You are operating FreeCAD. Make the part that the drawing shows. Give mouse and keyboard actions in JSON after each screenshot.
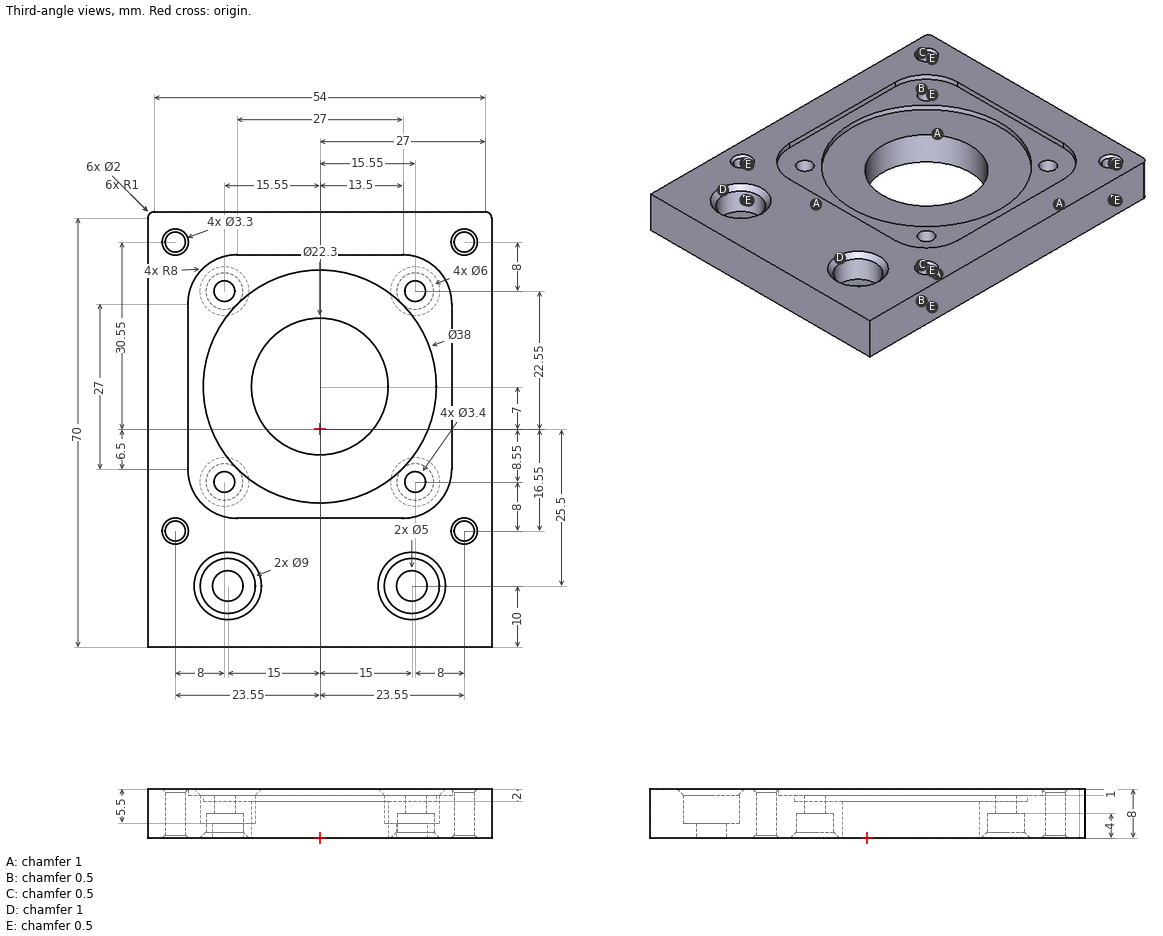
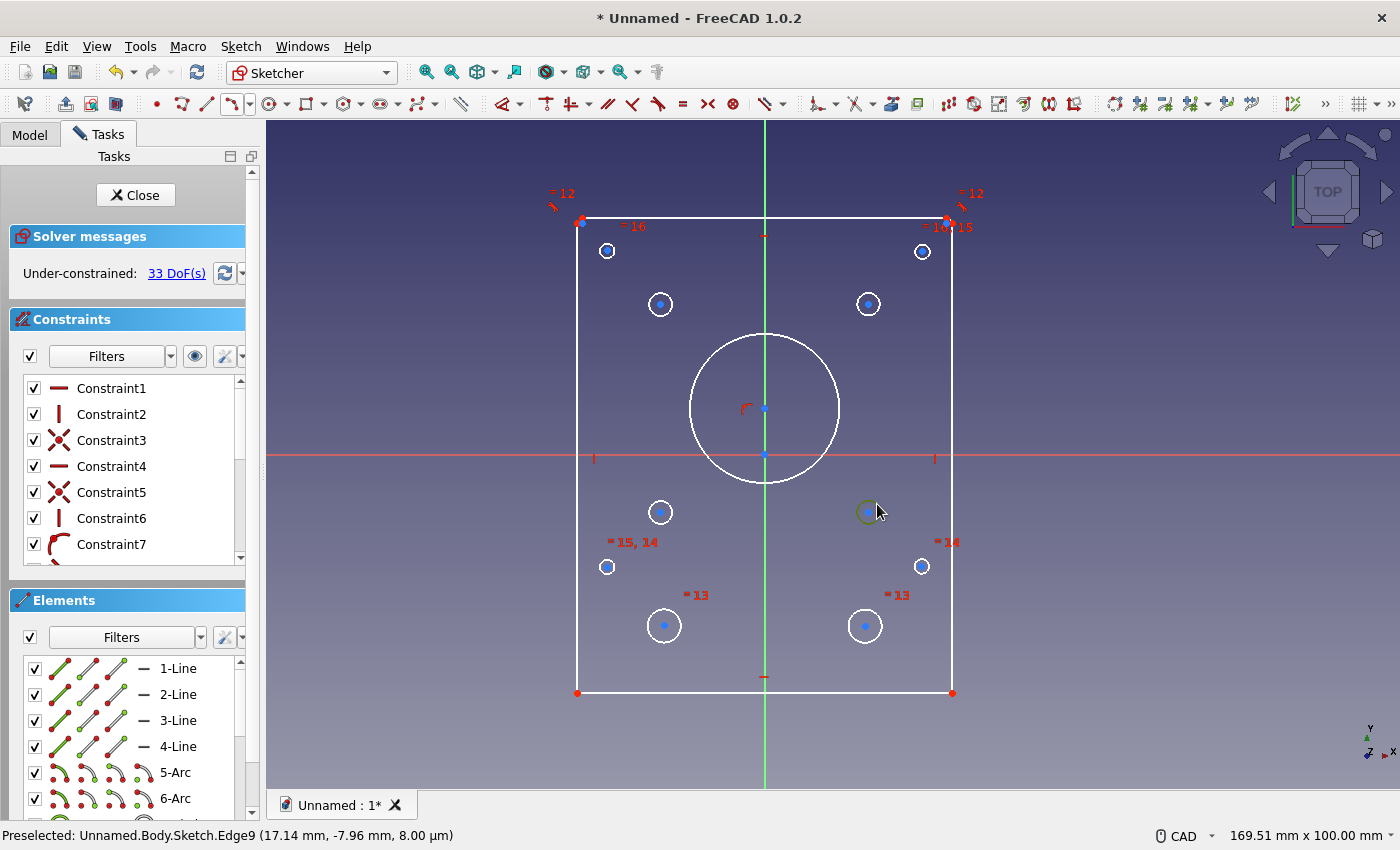
{"action": "left_click", "coordinate": [669, 504]}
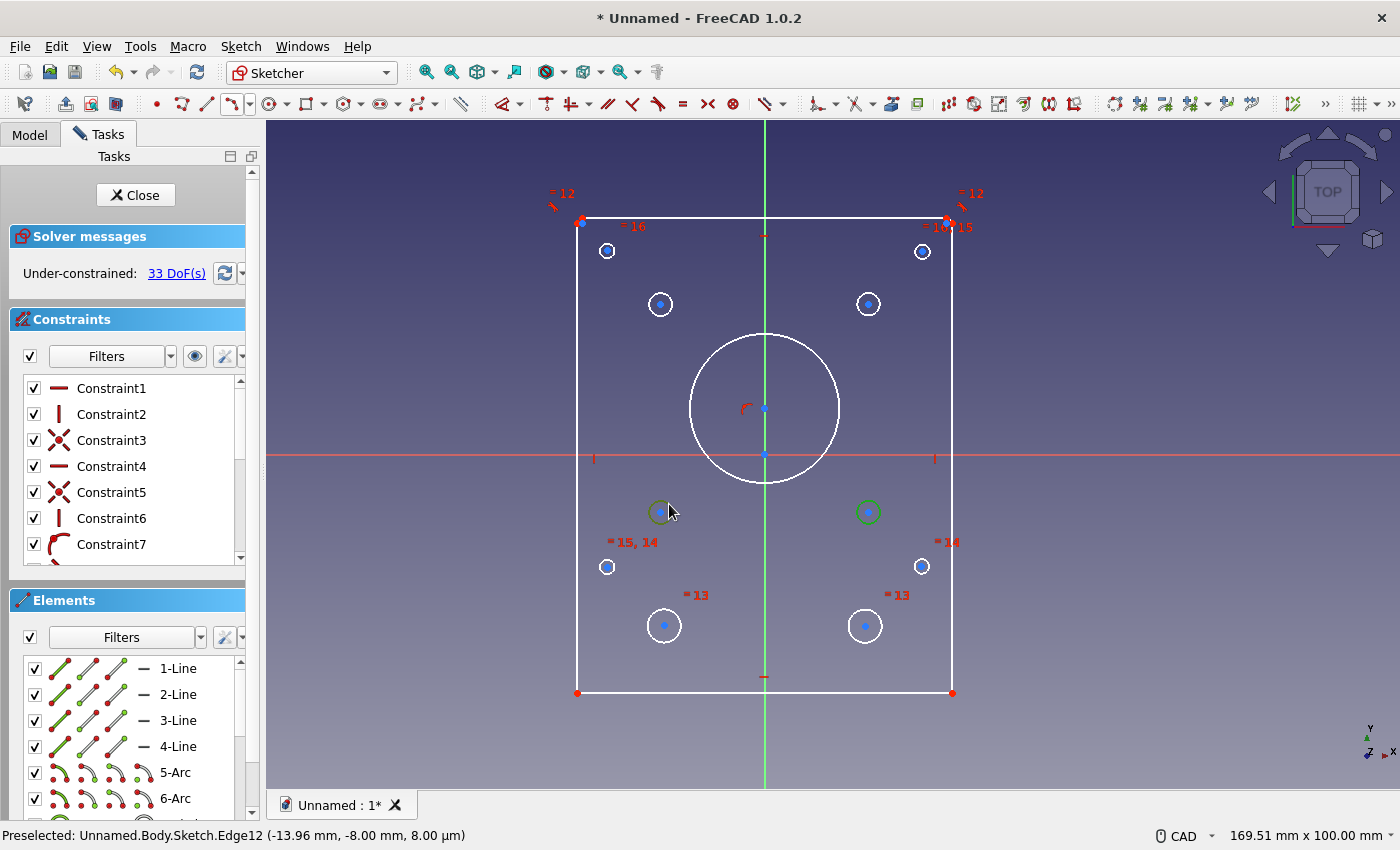
{"action": "scroll", "coordinate": [876, 296], "scroll_direction": "up", "scroll_amount": 2}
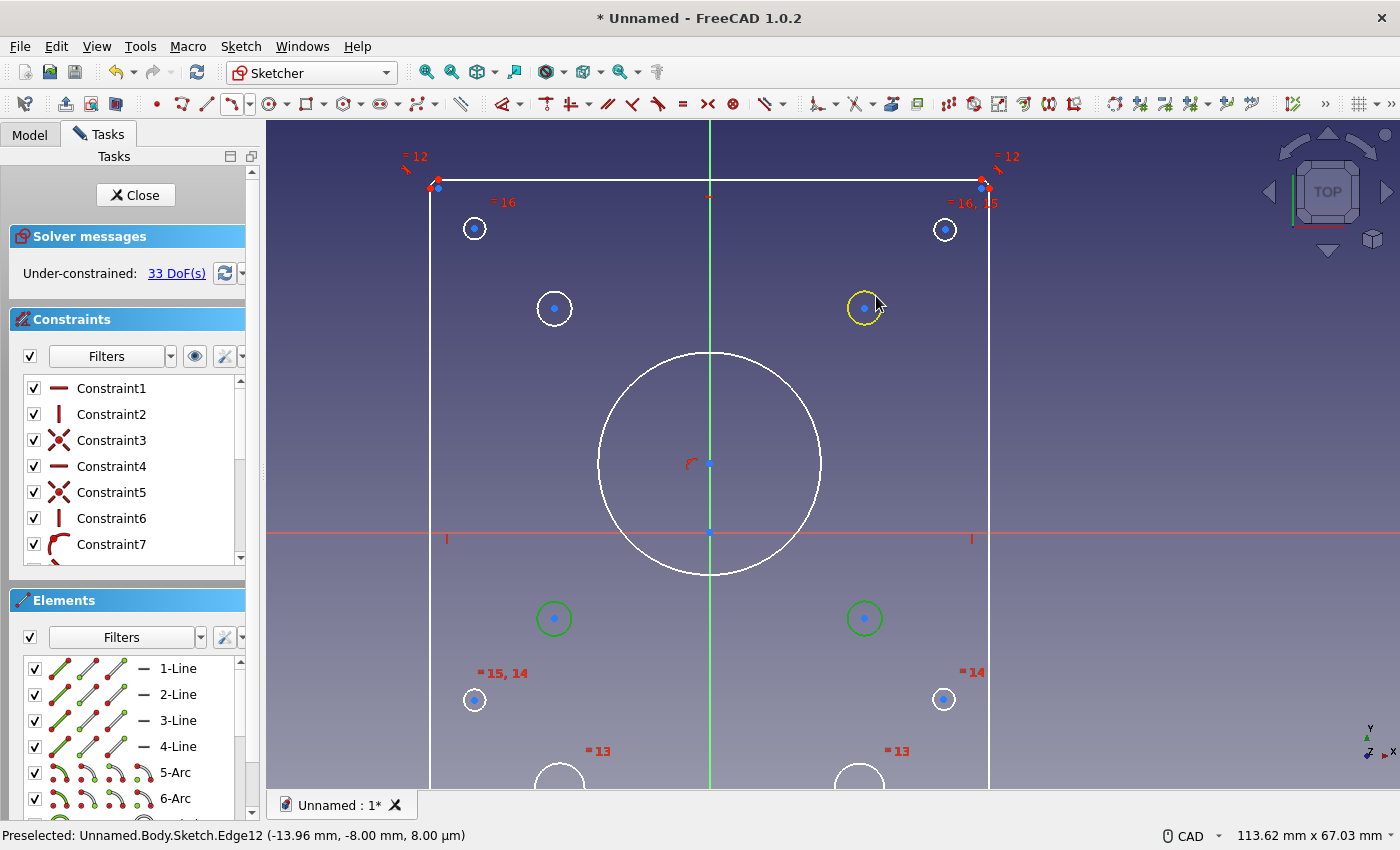
{"action": "left_click", "coordinate": [876, 296]}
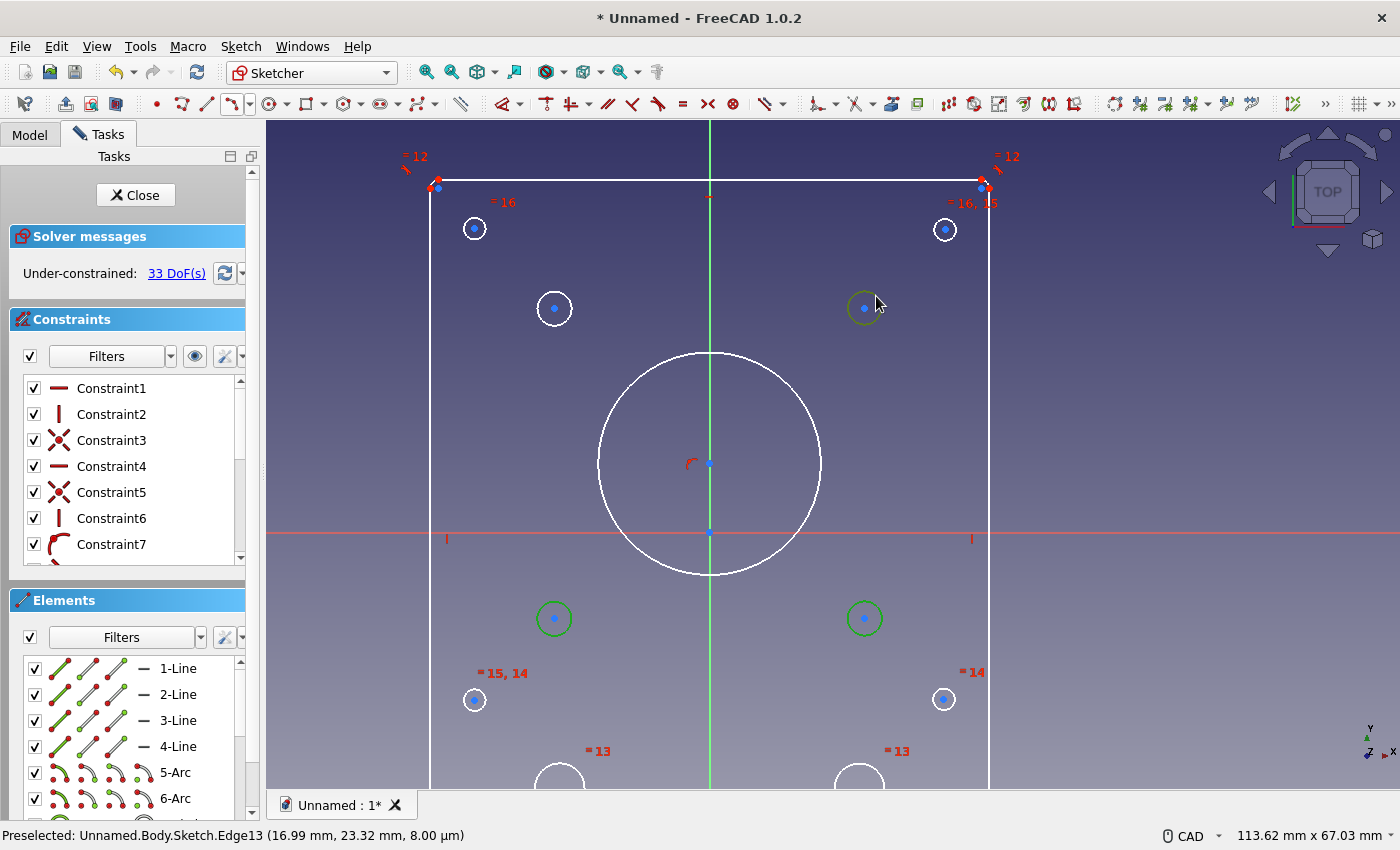
{"action": "left_click", "coordinate": [567, 297]}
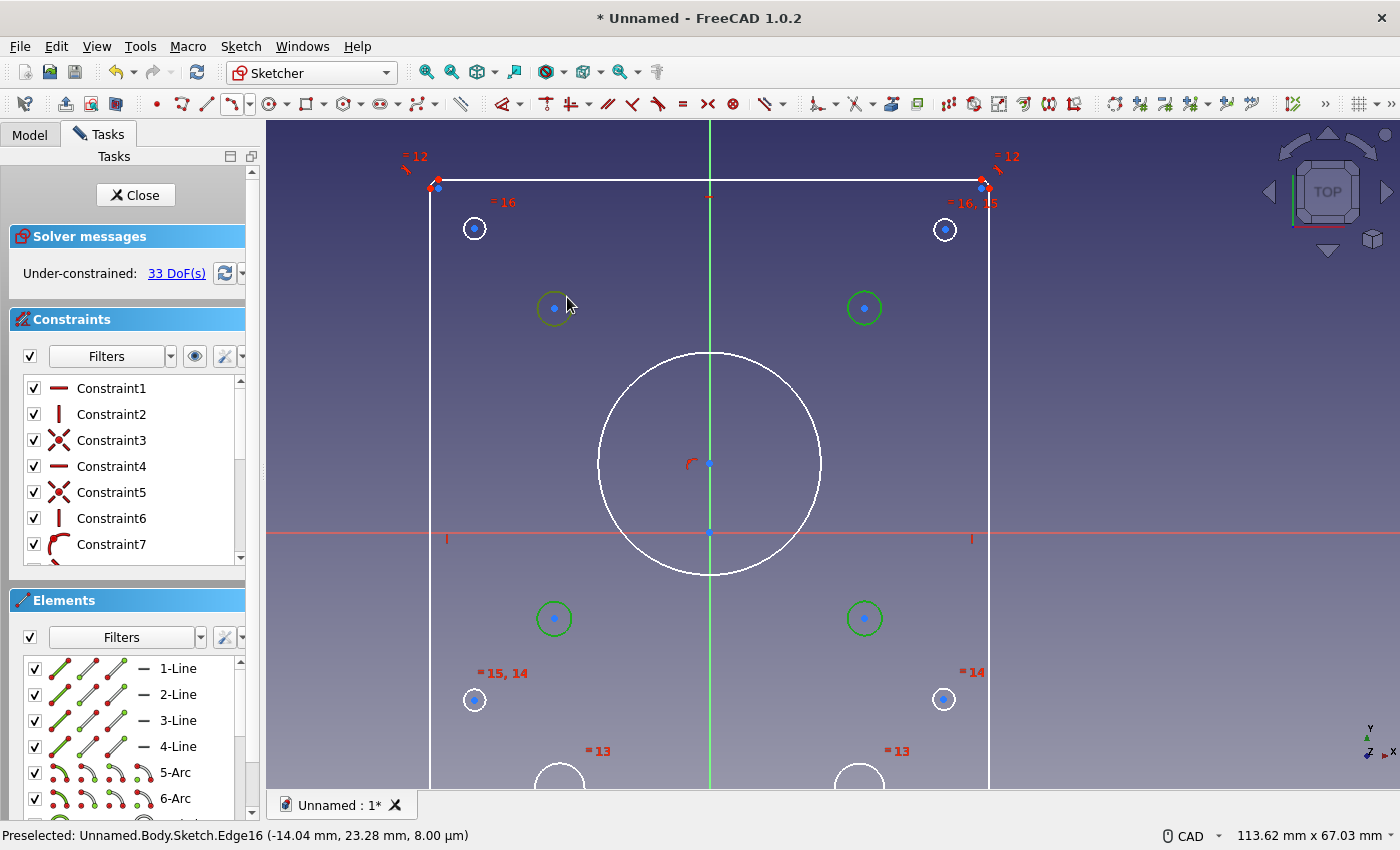
{"action": "left_click", "coordinate": [683, 104]}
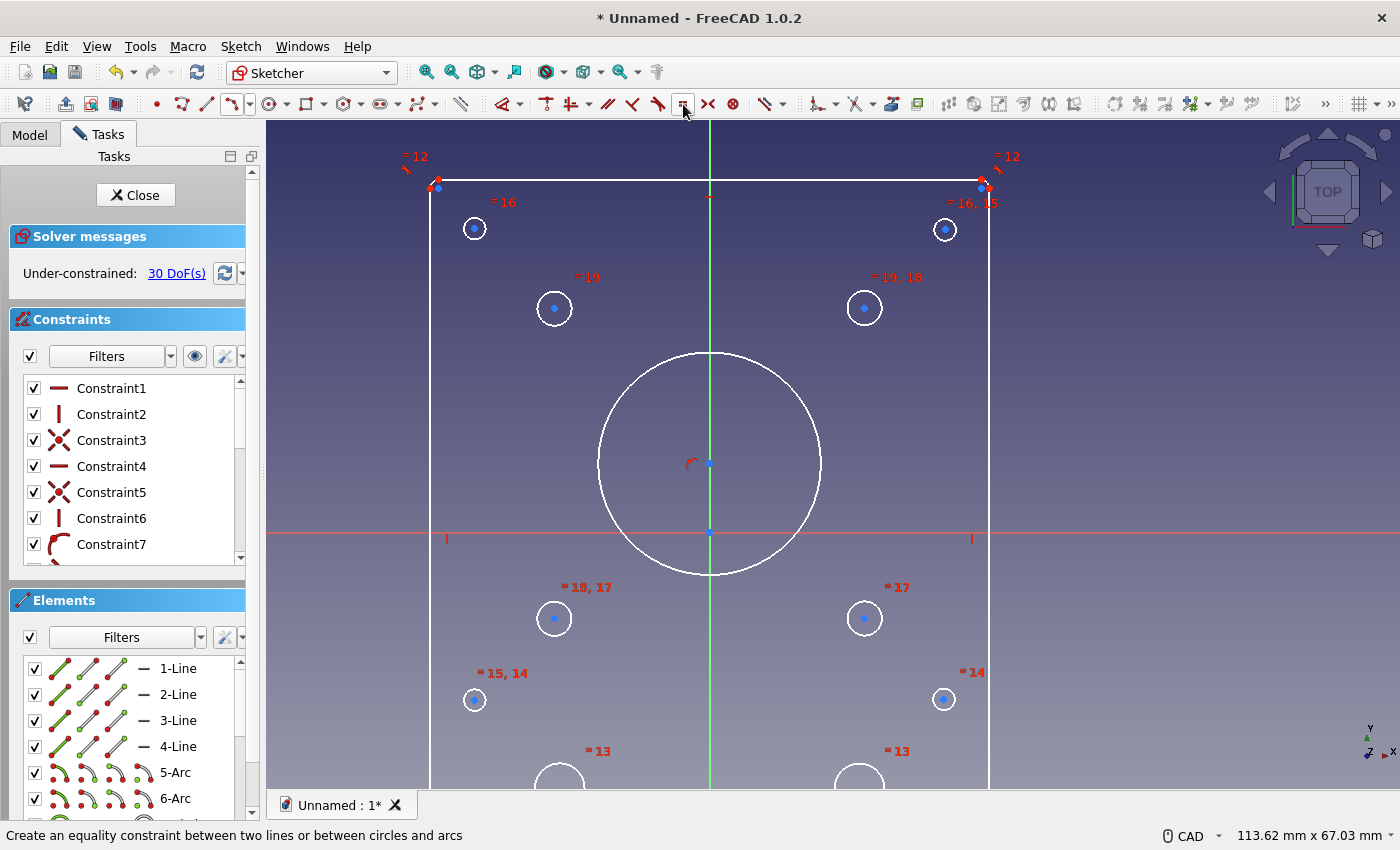
{"action": "key", "text": "d"}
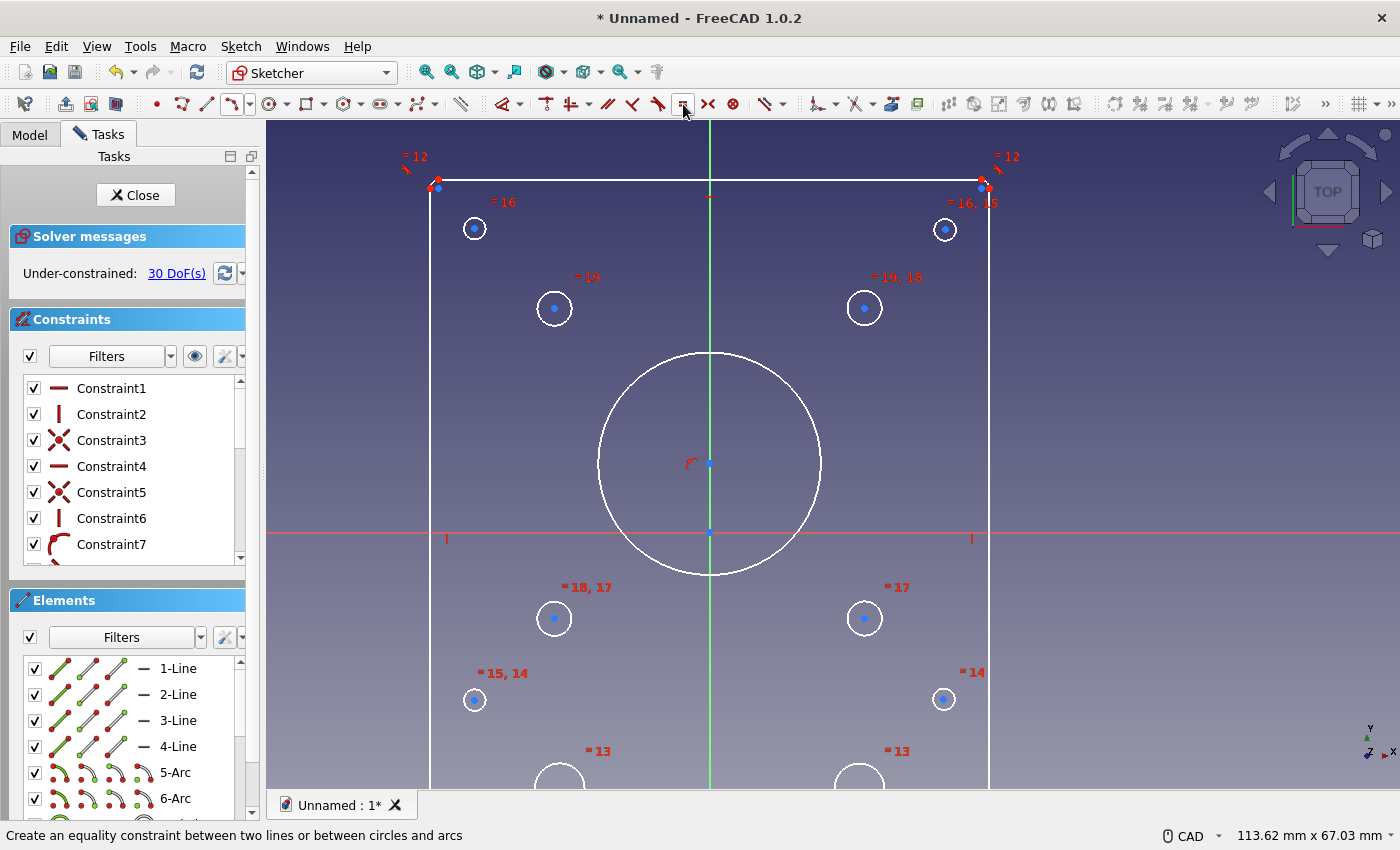
{"action": "scroll", "coordinate": [433, 182], "scroll_direction": "up", "scroll_amount": 7}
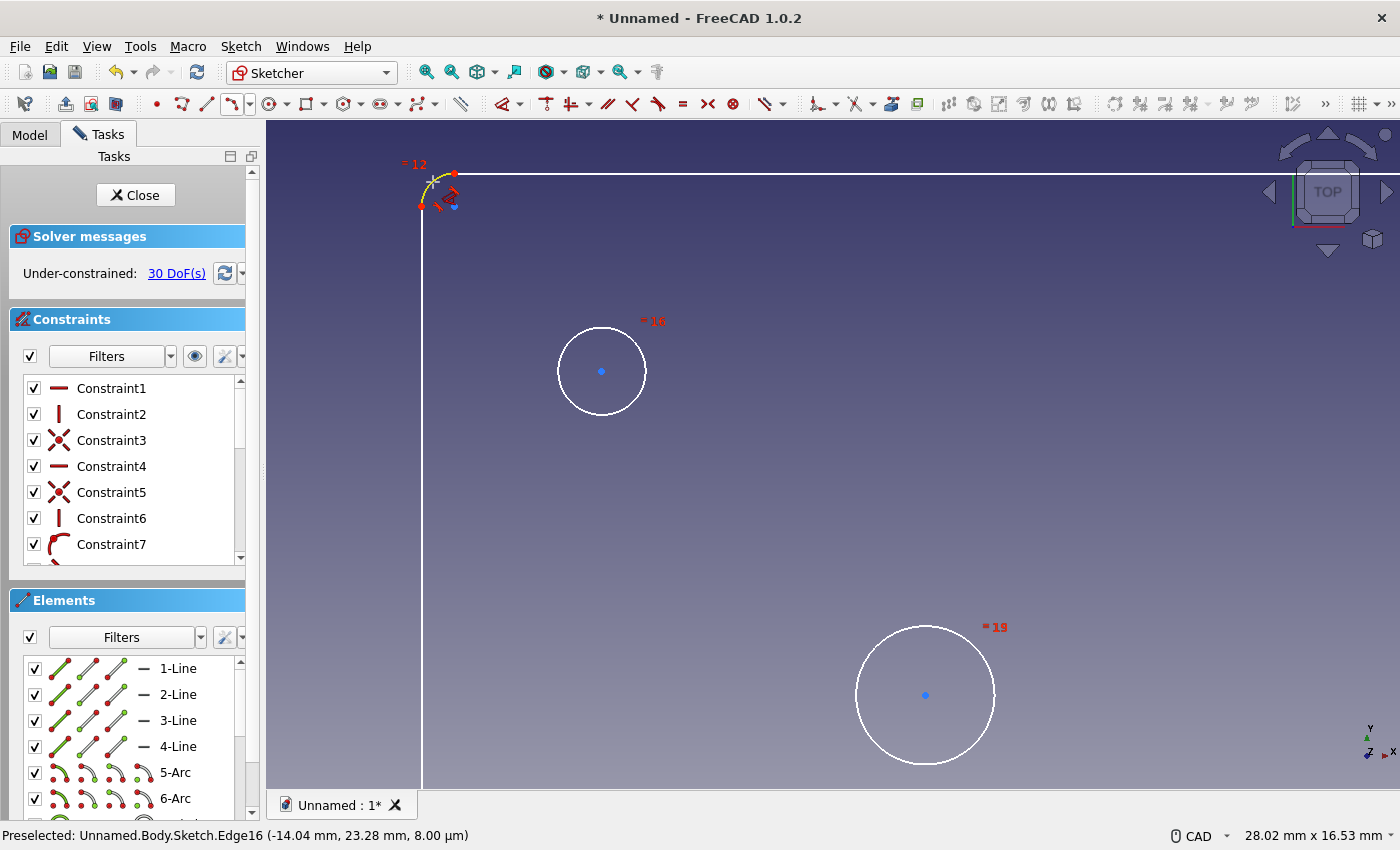
{"action": "left_click", "coordinate": [431, 183]}
{"action": "left_click", "coordinate": [408, 161]}